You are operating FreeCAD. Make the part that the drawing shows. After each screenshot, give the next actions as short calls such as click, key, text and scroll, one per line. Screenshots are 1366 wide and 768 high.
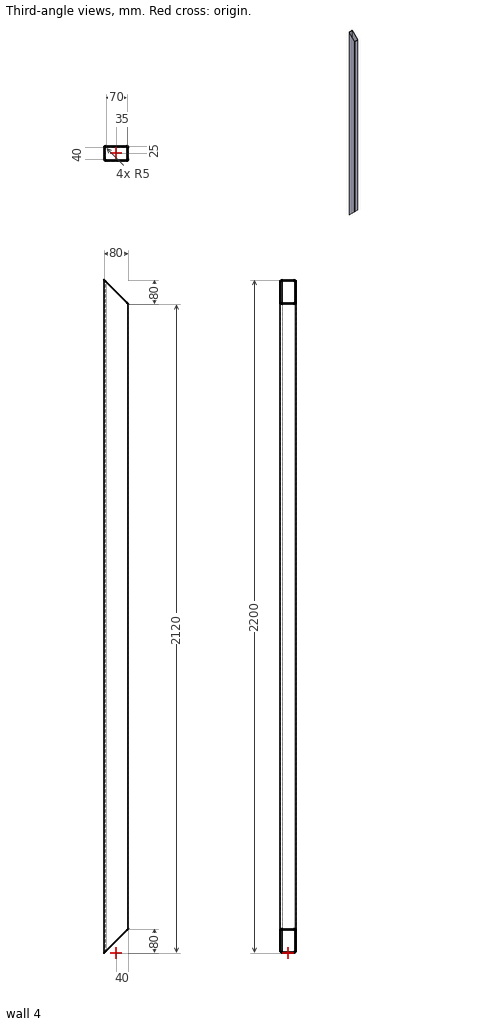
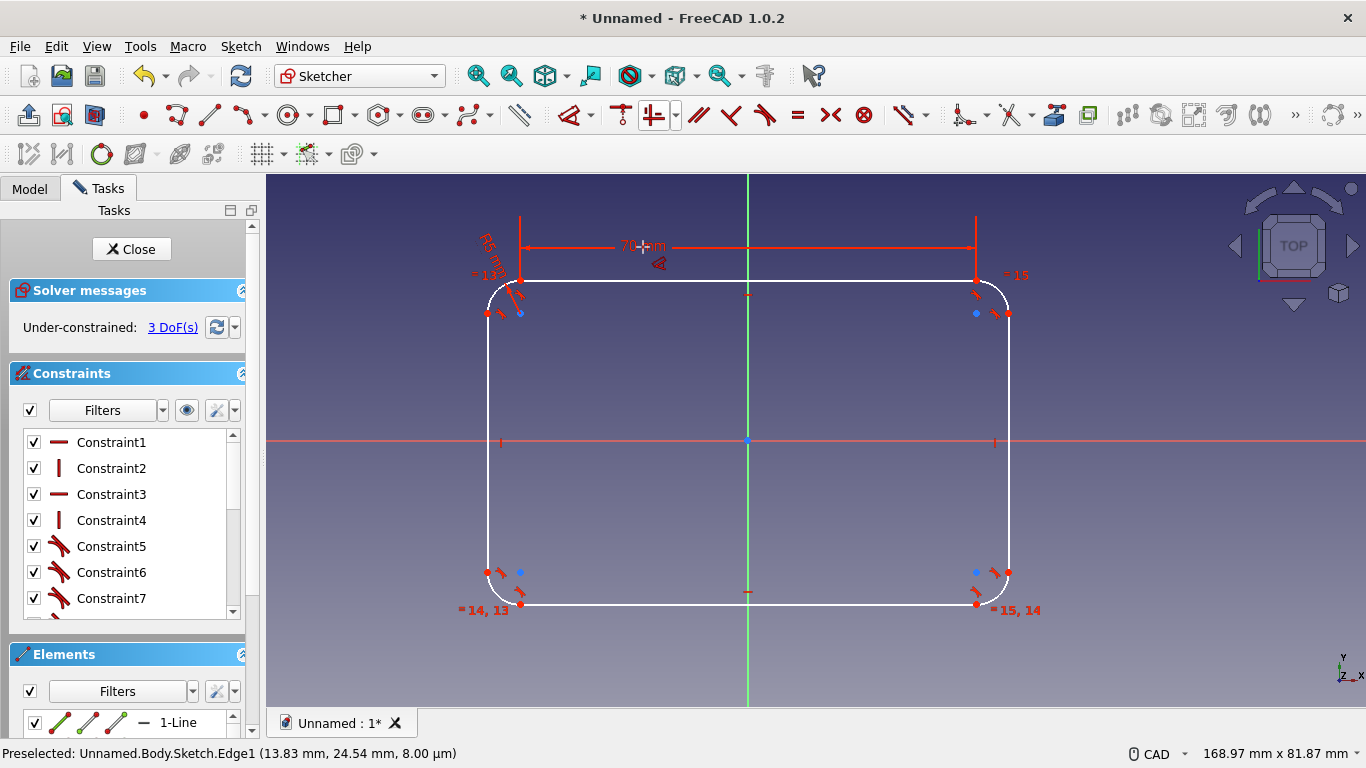
click(488, 391)
click(454, 383)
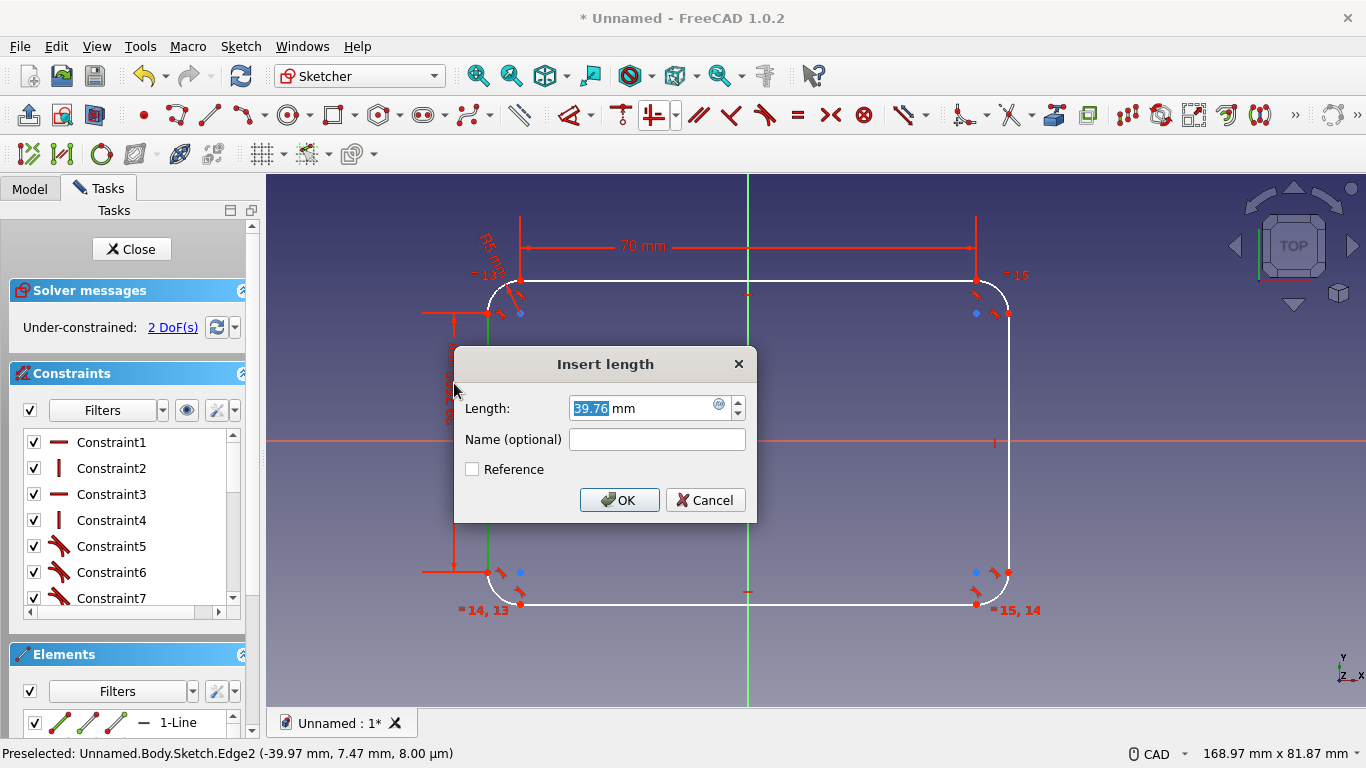
text(40)
key(Return)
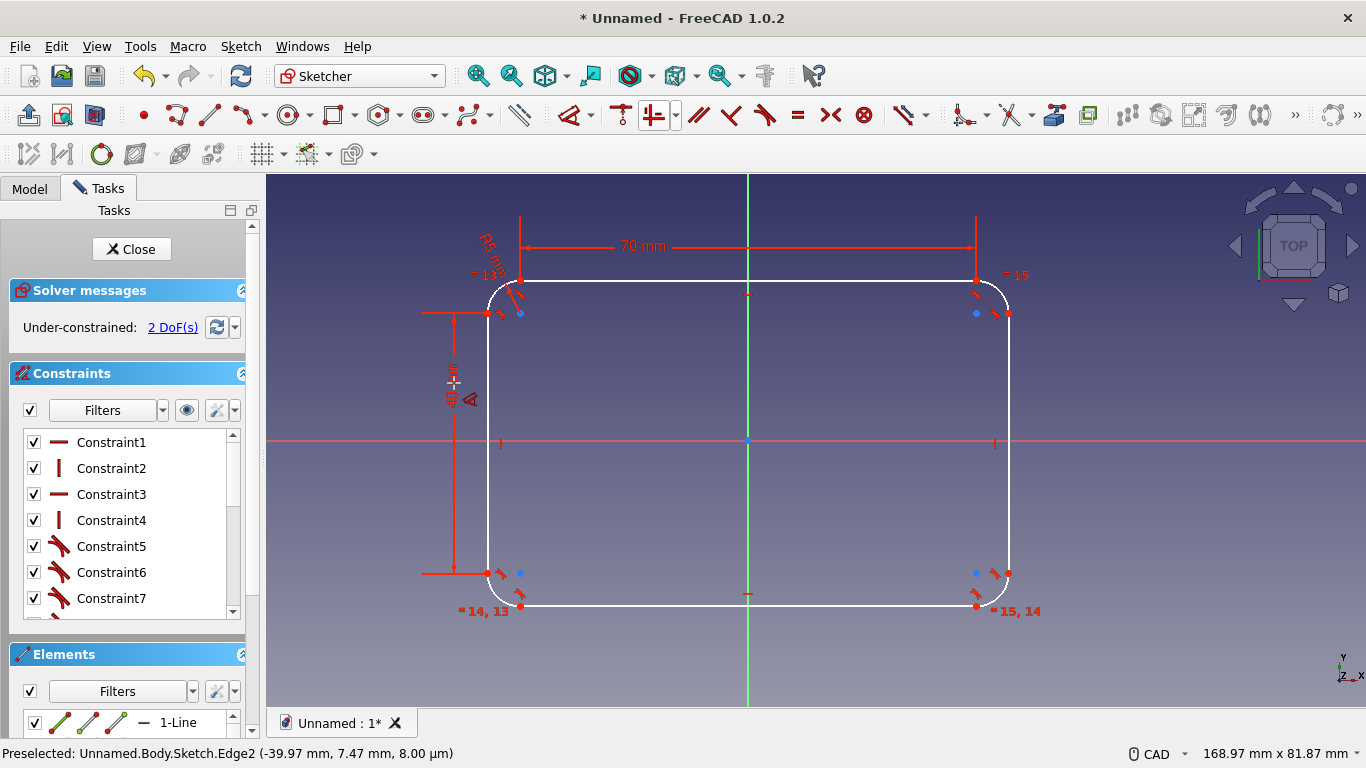
click(976, 281)
click(862, 247)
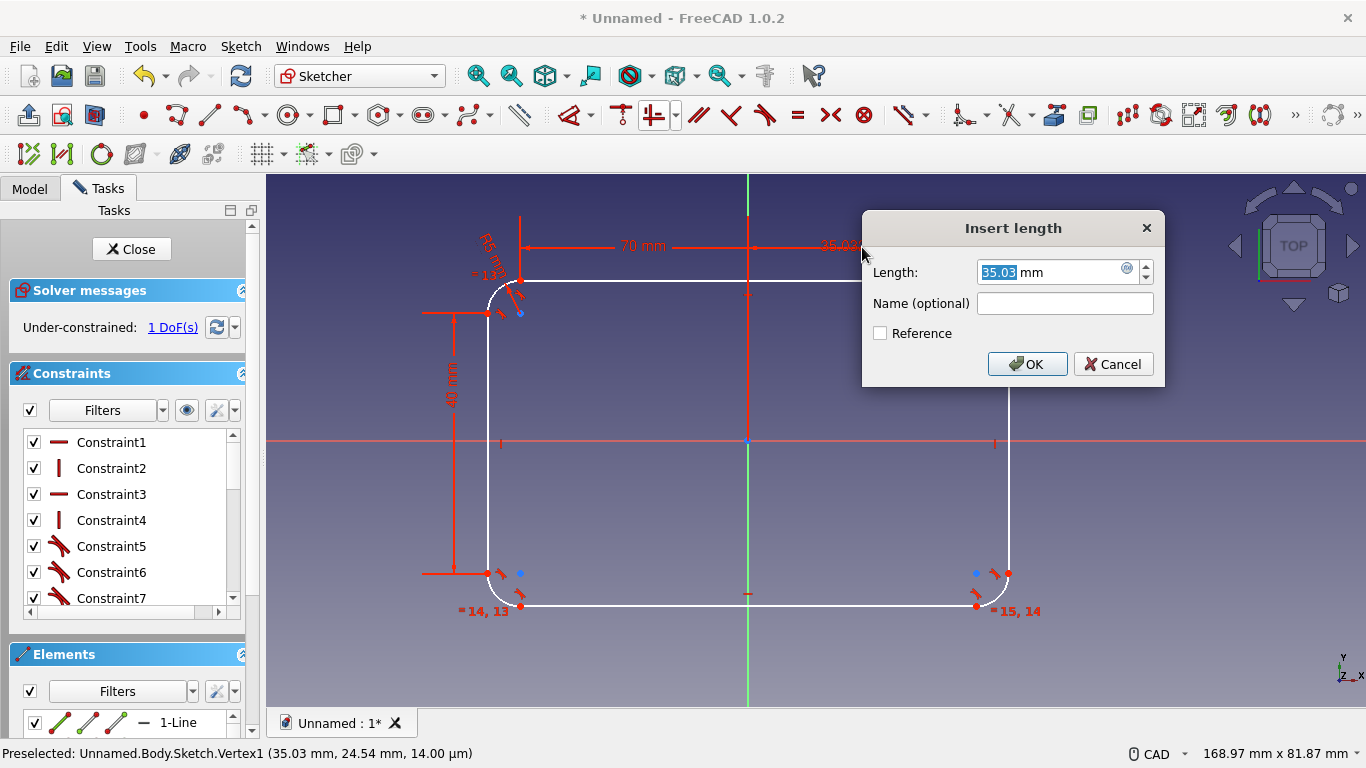
text(35)
key(Return)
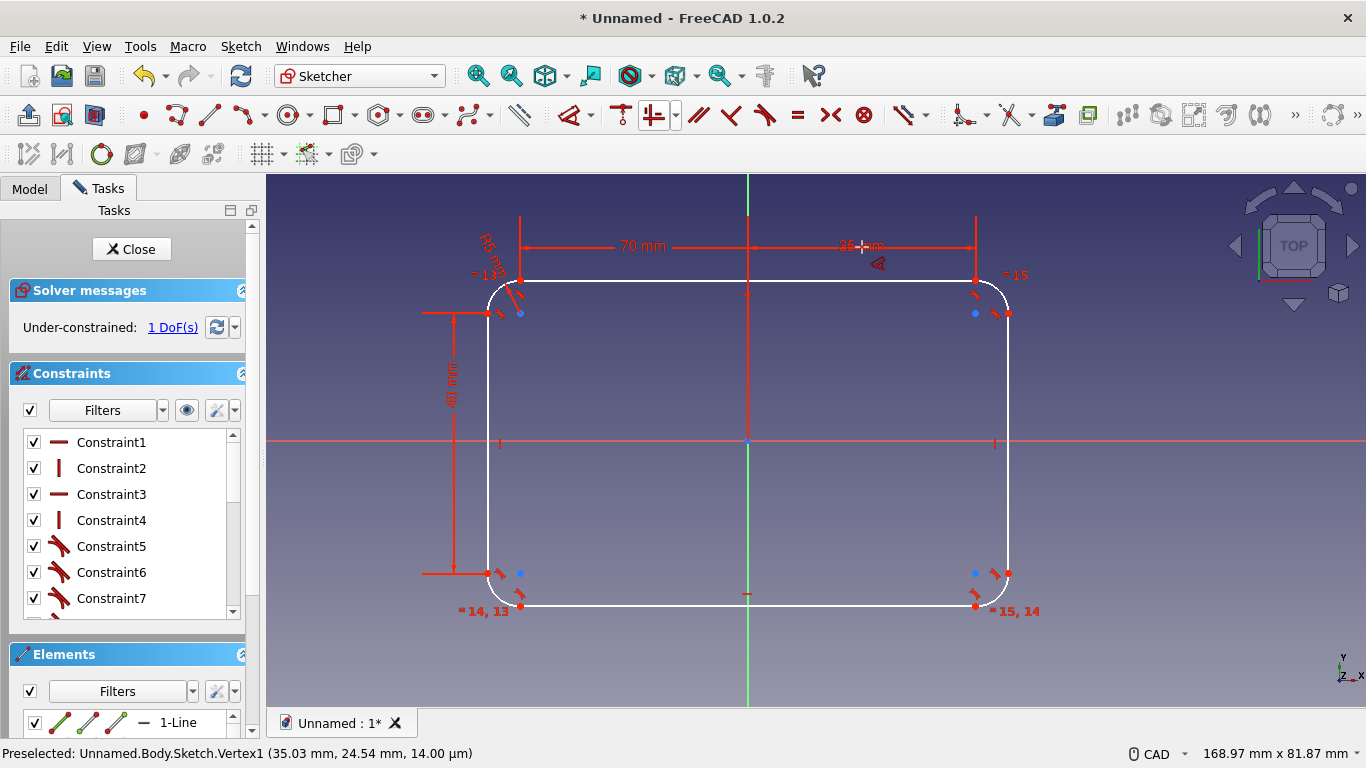
click(976, 281)
click(714, 361)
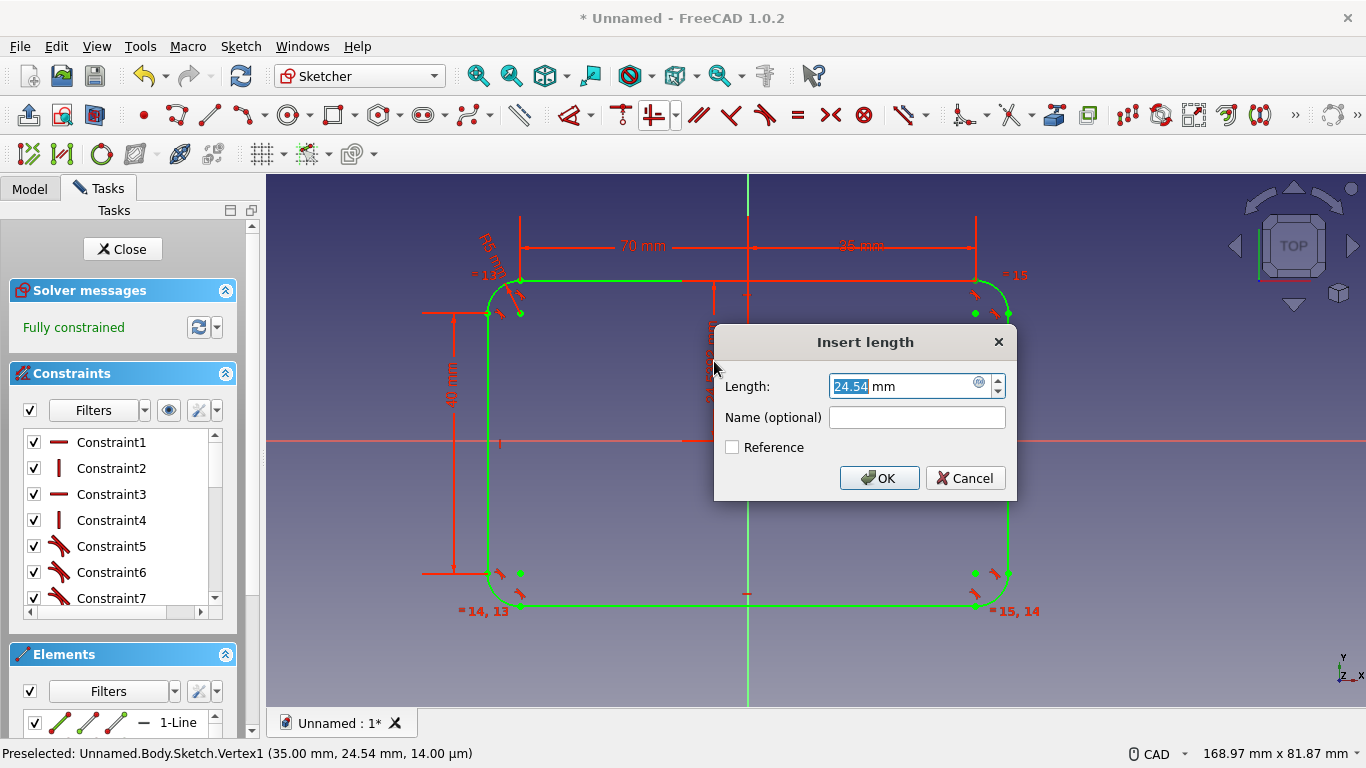
text(25)
key(Return)
key(Escape)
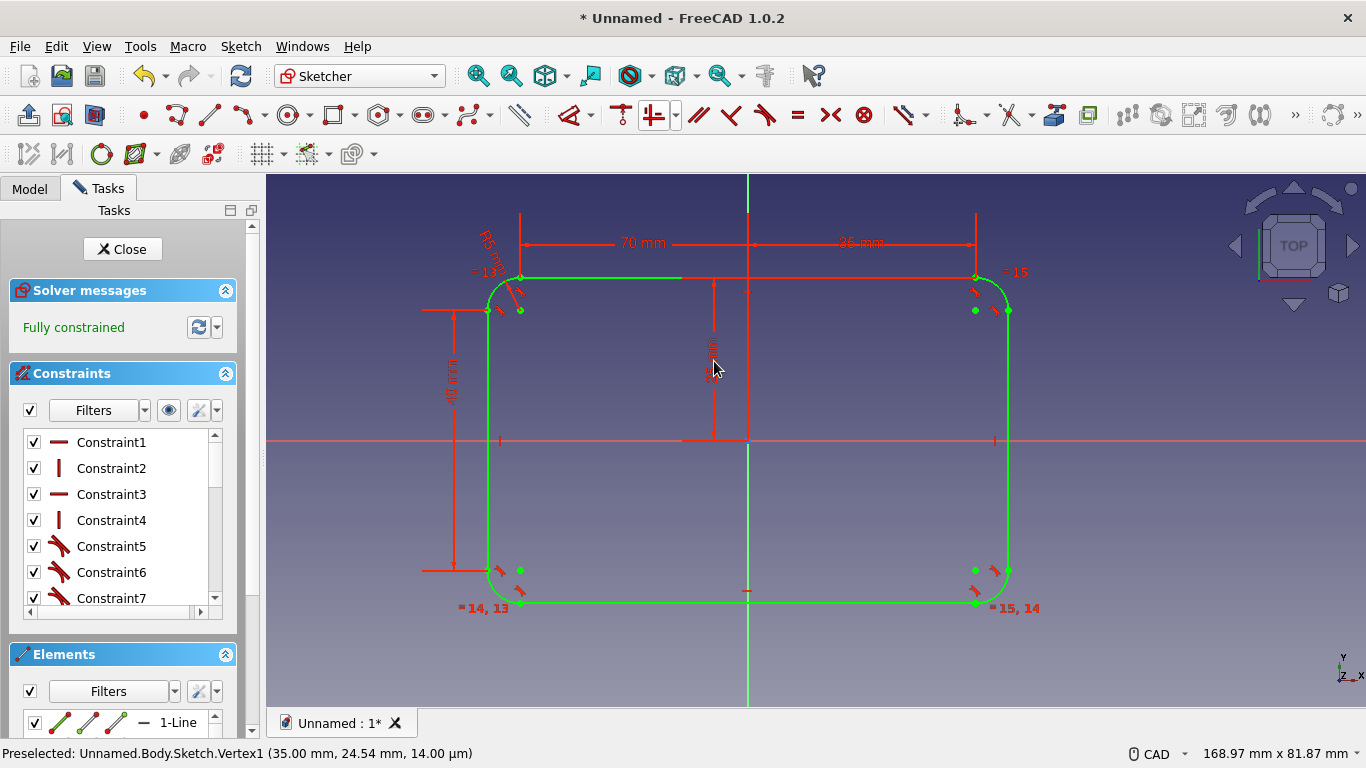
click(123, 249)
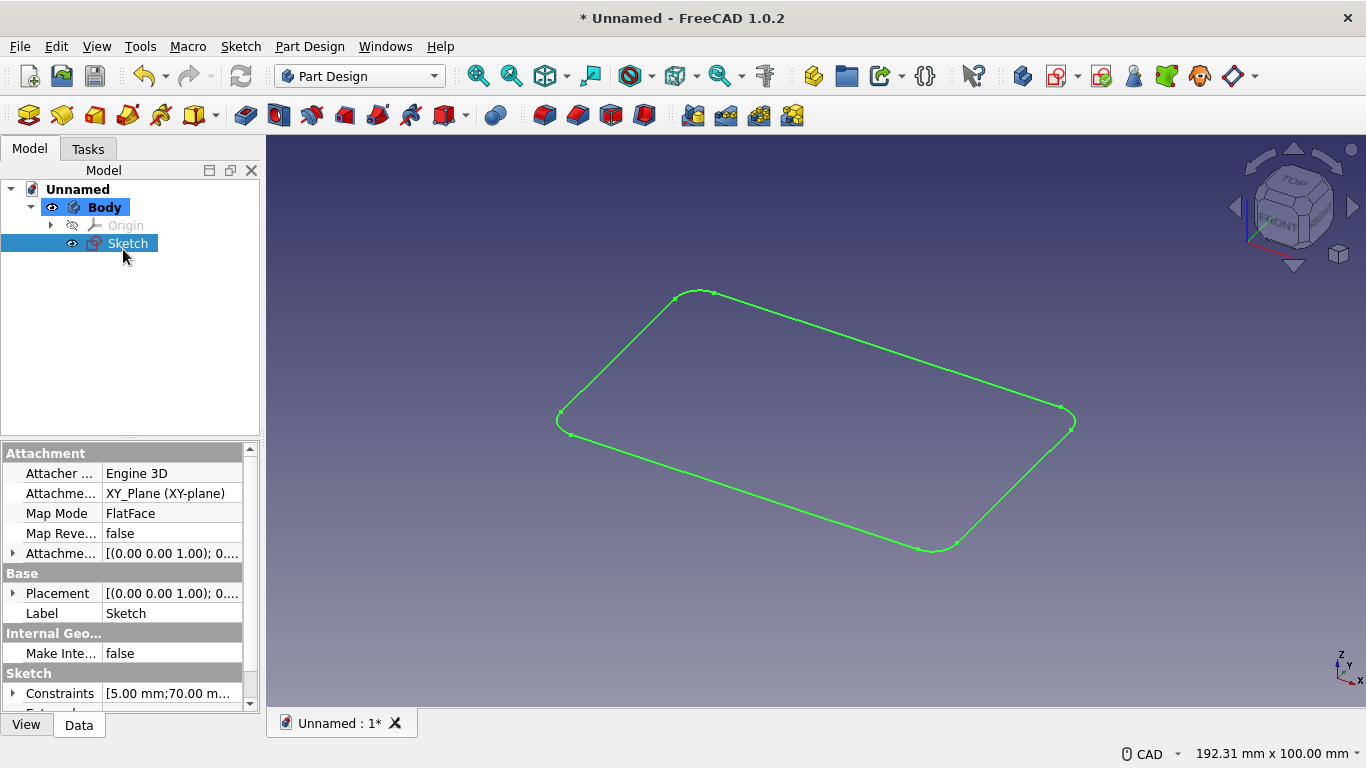
click(29, 116)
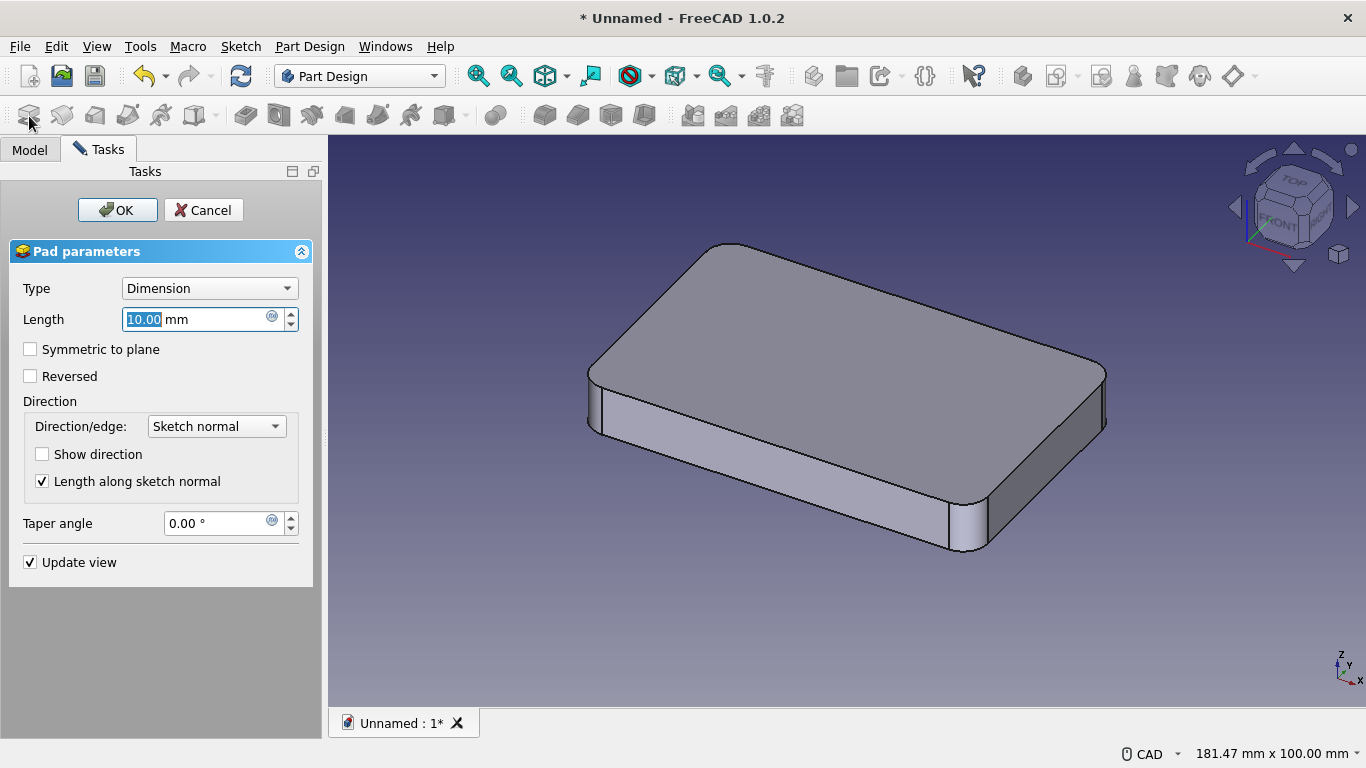
text(2200)
key(Tab)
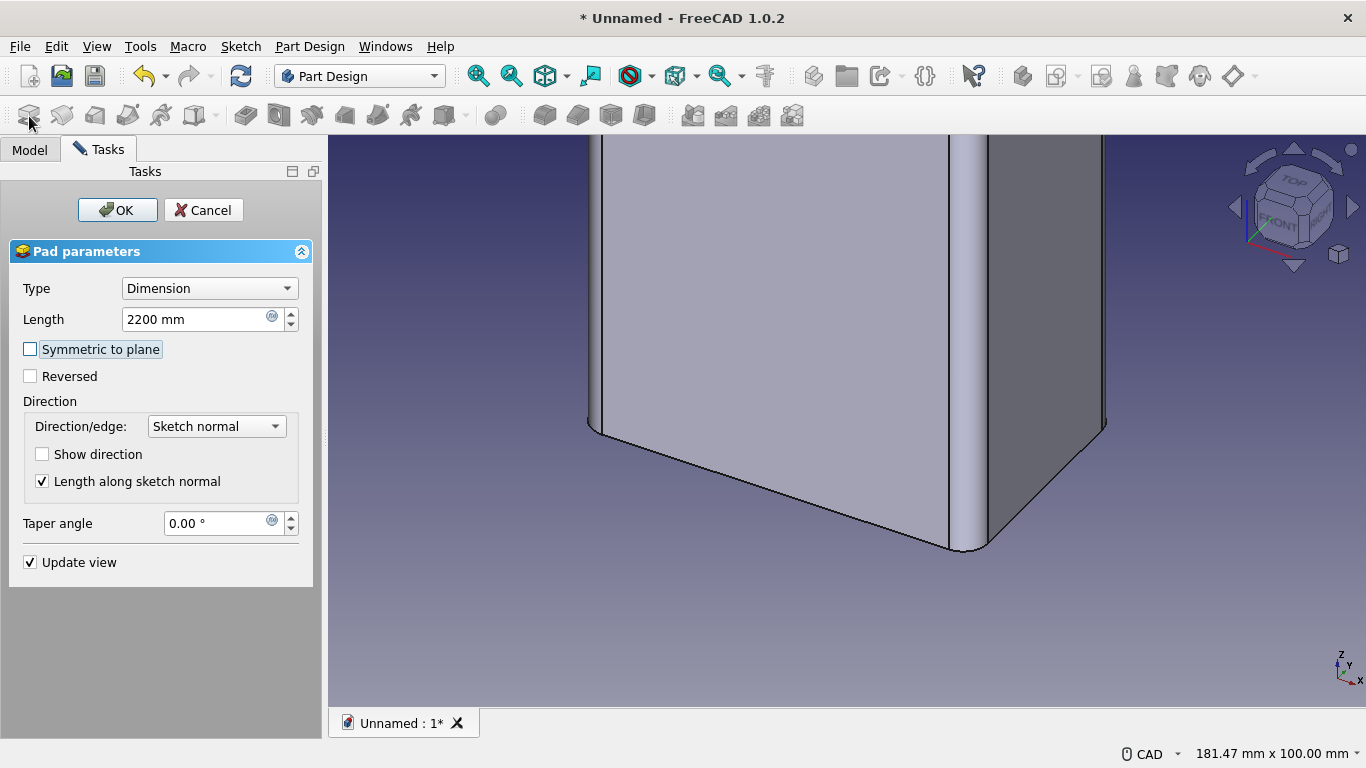
click(118, 210)